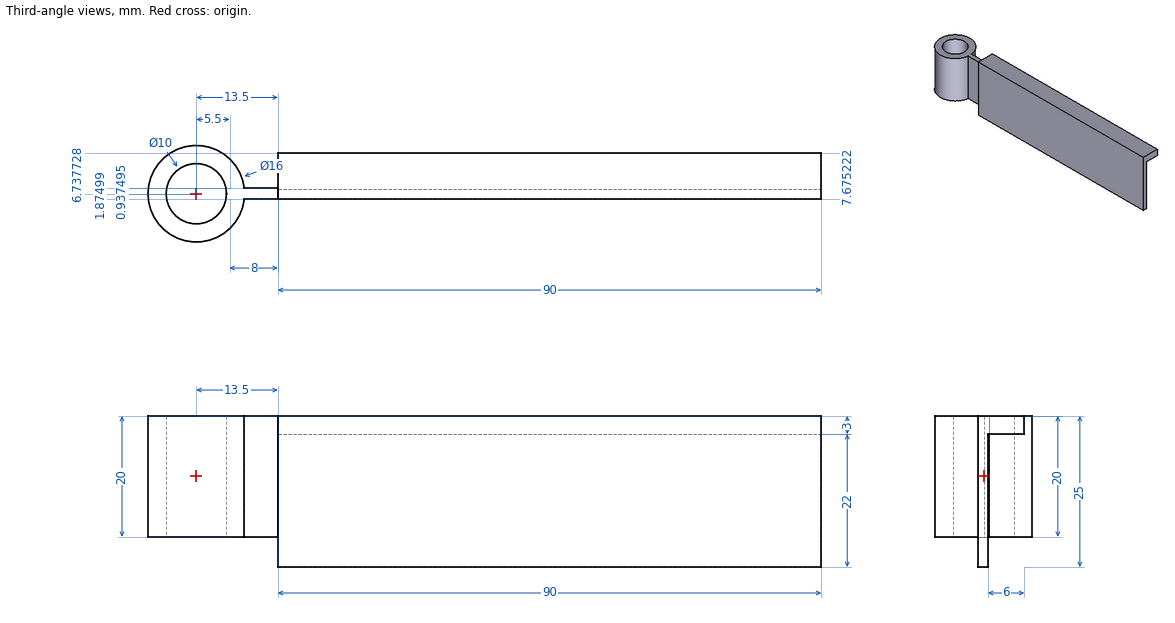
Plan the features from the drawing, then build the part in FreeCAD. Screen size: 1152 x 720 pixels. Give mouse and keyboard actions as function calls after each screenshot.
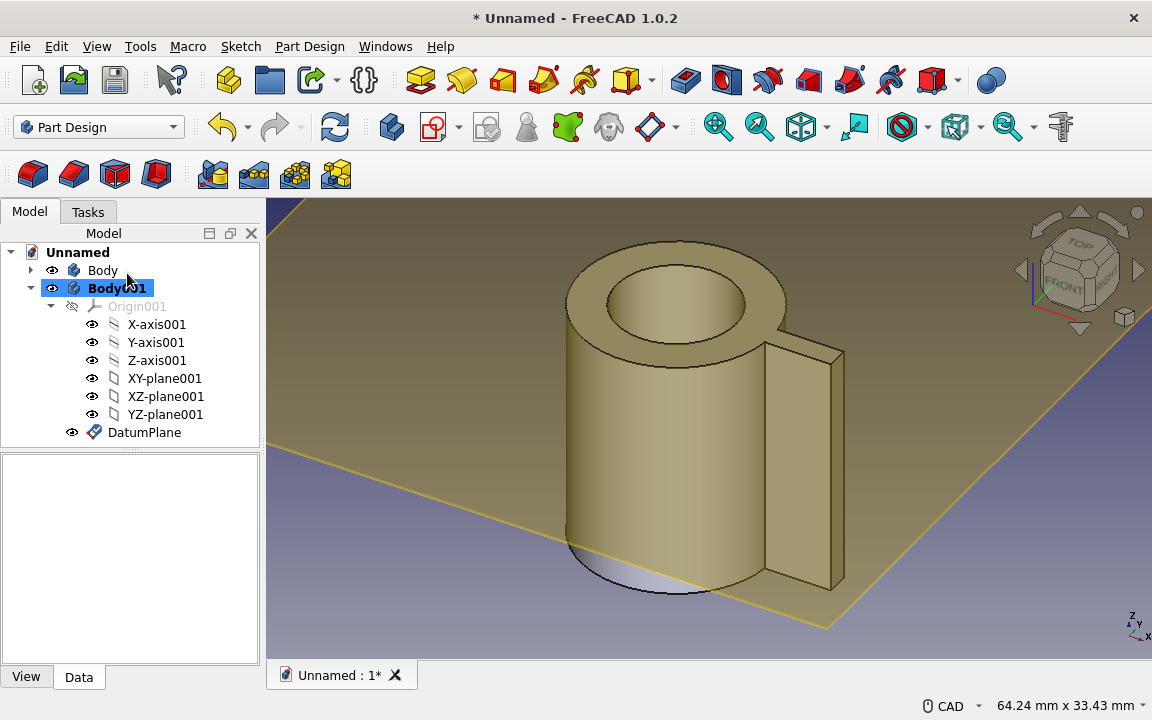
click(117, 432)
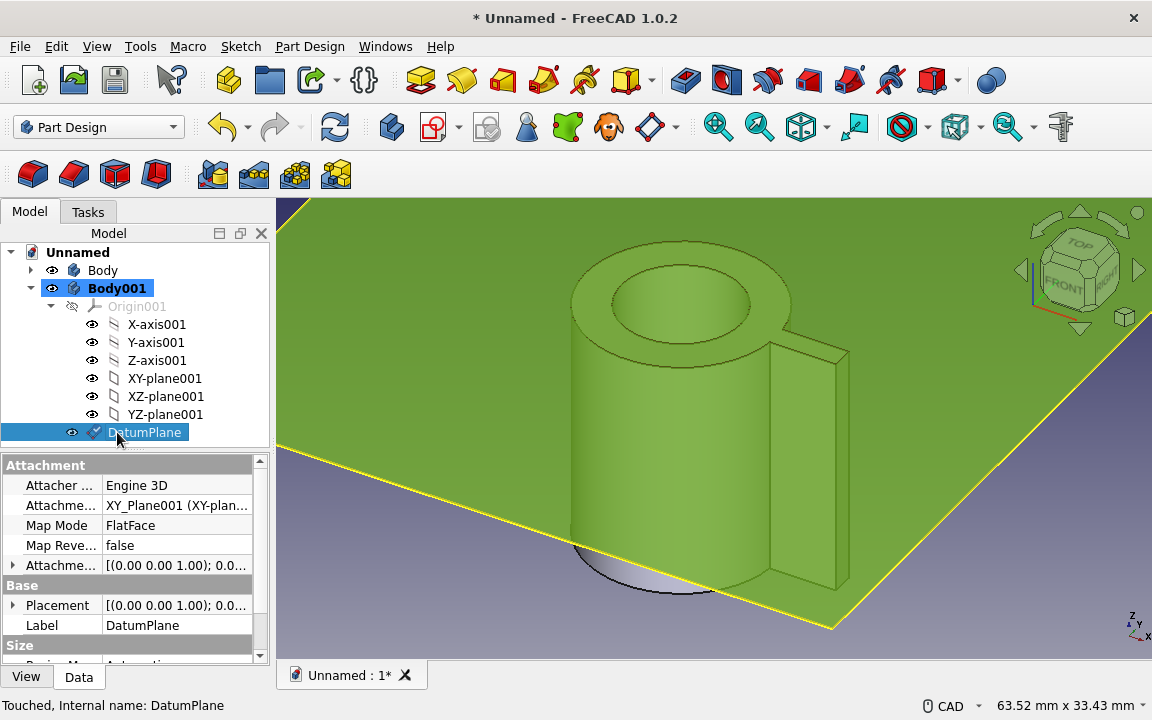
click(432, 128)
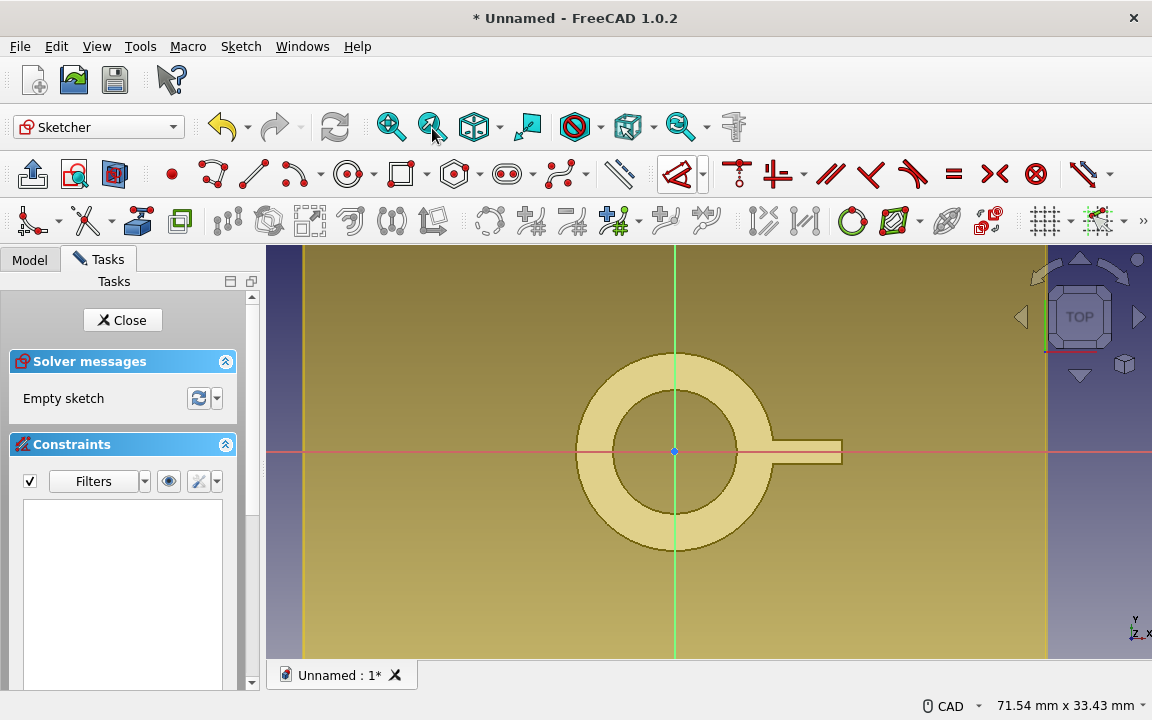
scroll(294, 473, down, 5)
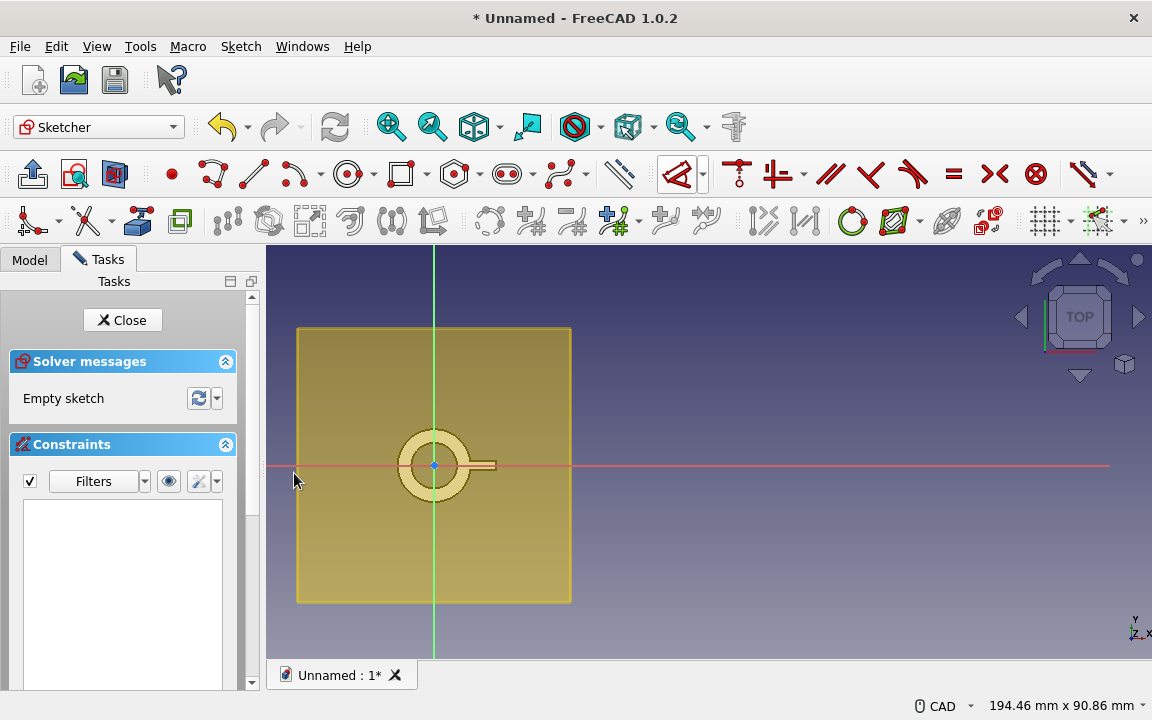
click(400, 174)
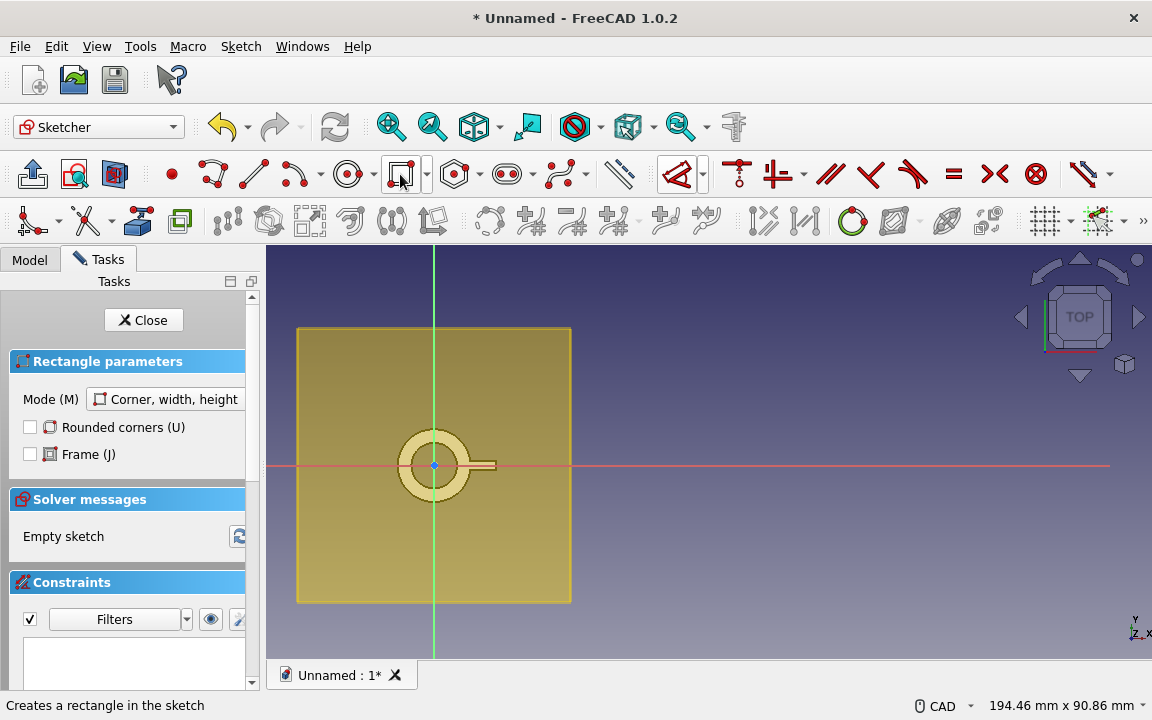
click(496, 435)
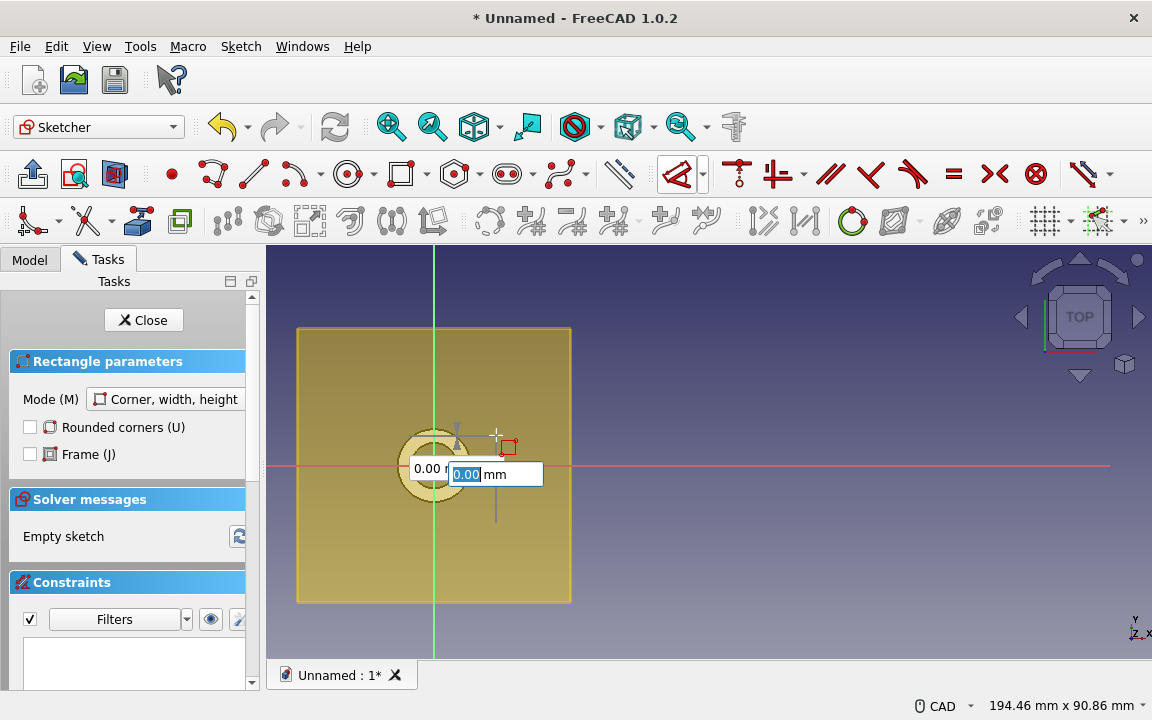
scroll(906, 470, up, 7)
move(903, 468)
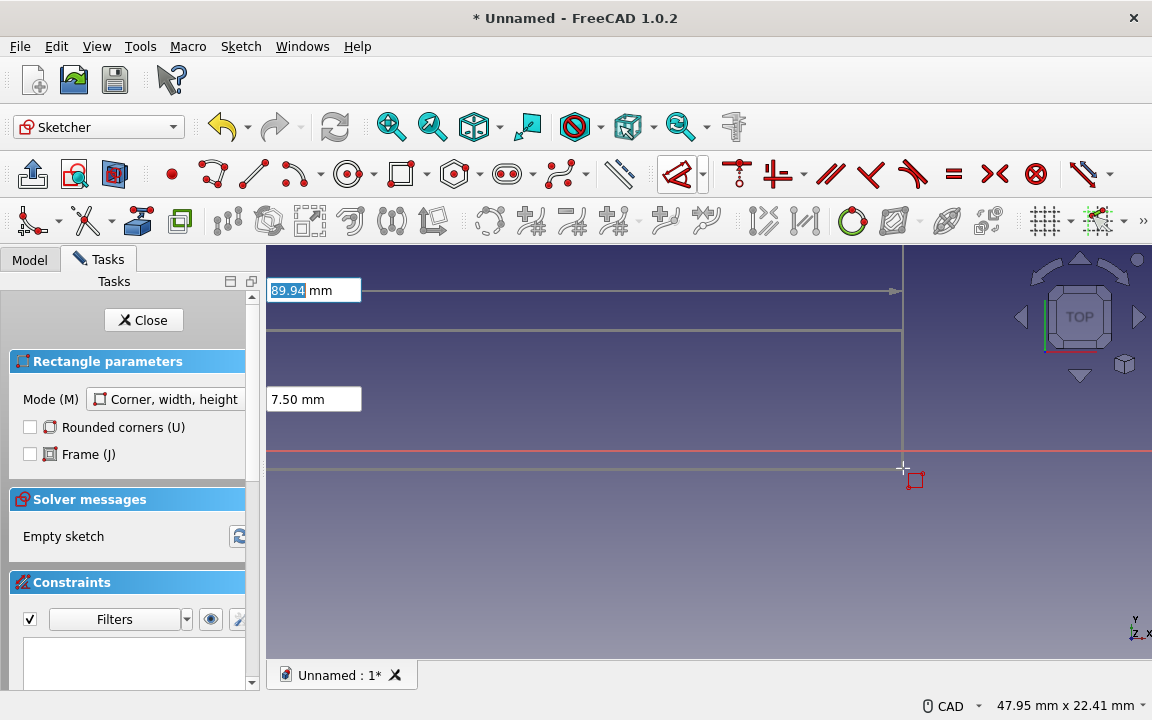
text(90)
key(Tab)
text(7.675222)
key(Return)
key(Escape)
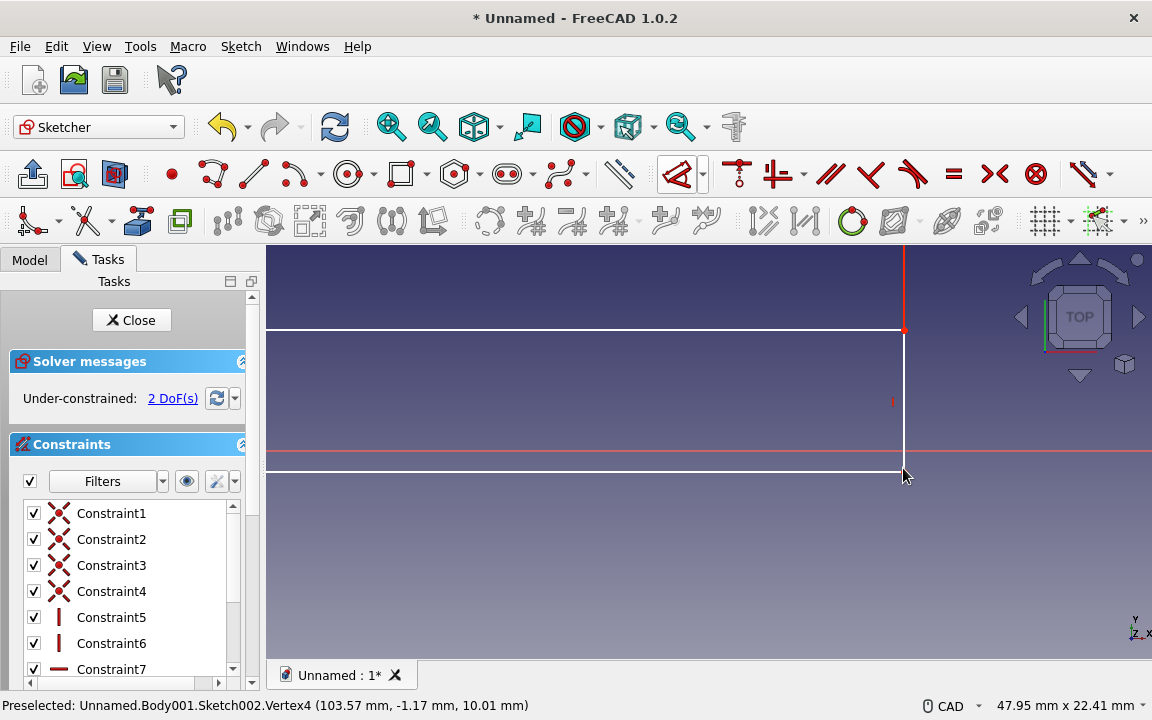
scroll(868, 470, down, 7)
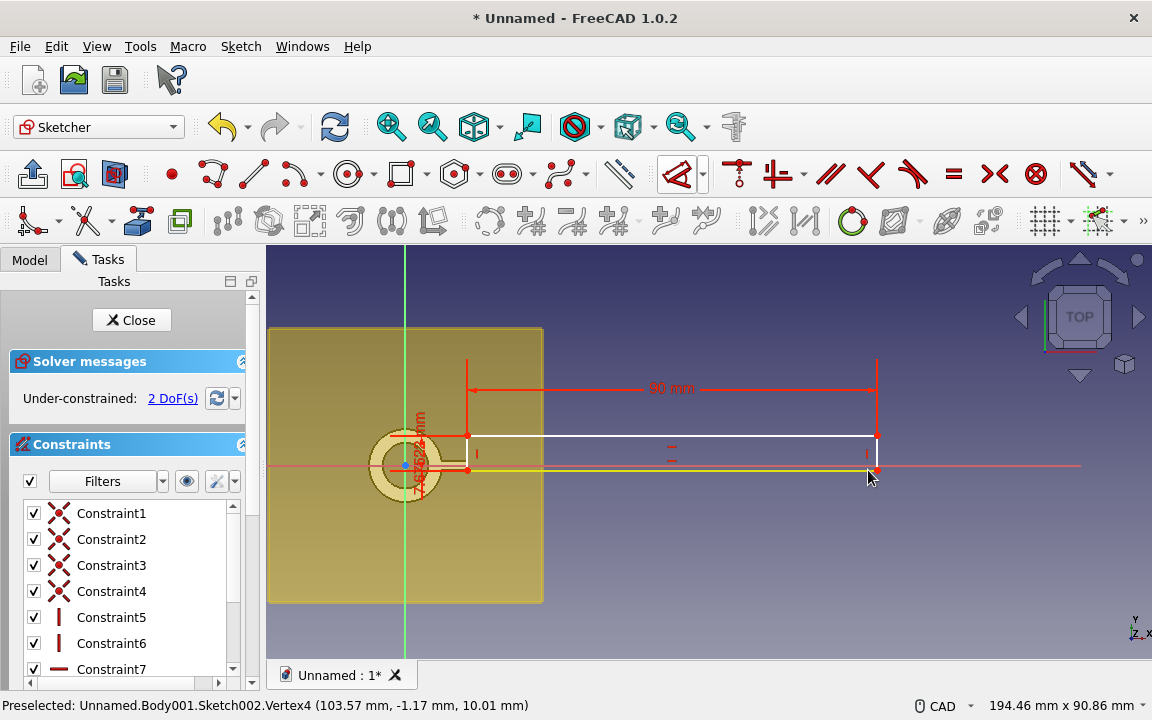
click(467, 436)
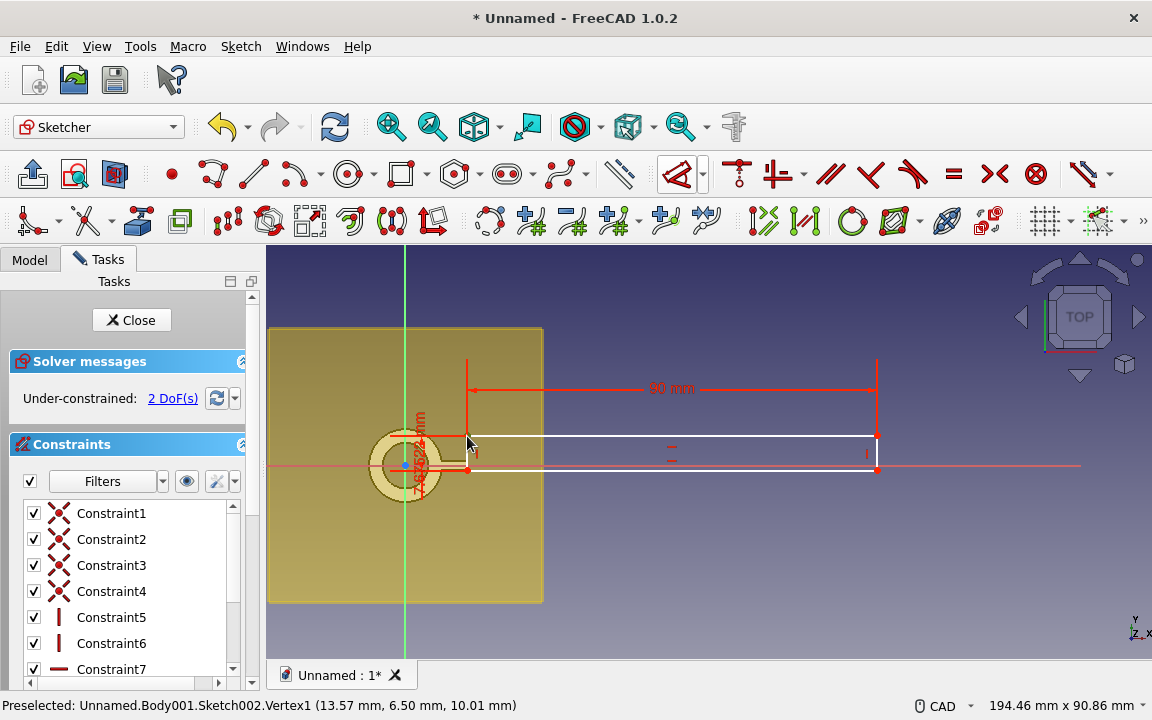
click(702, 174)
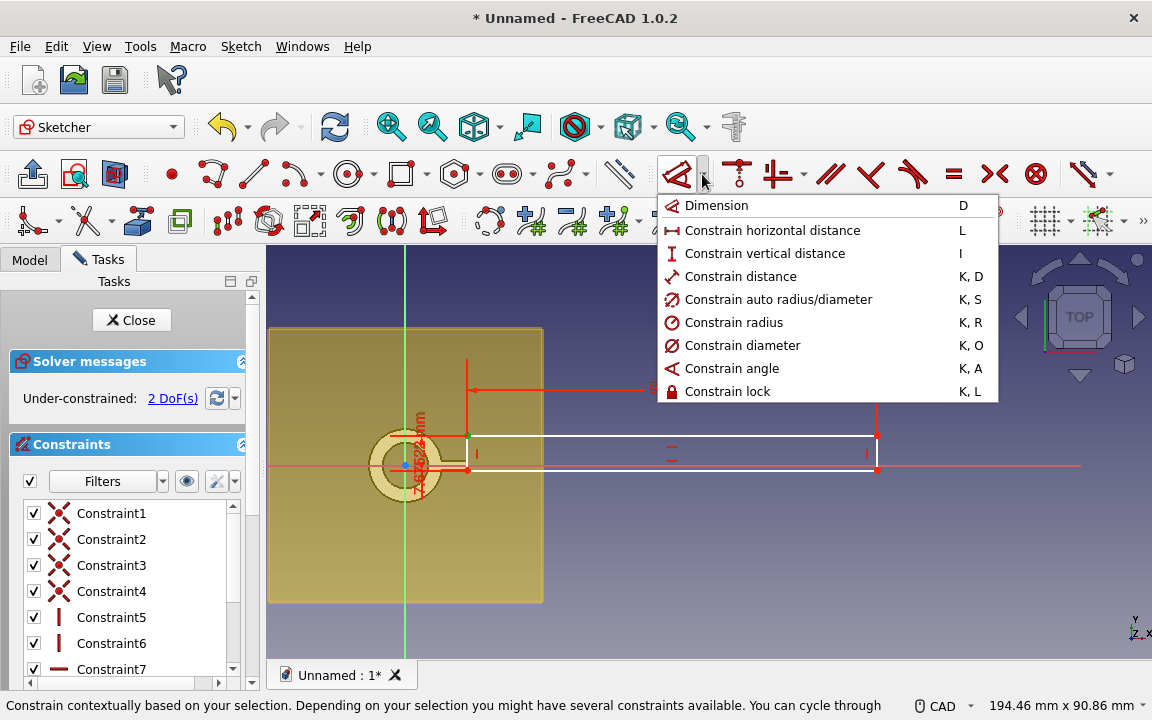
click(828, 230)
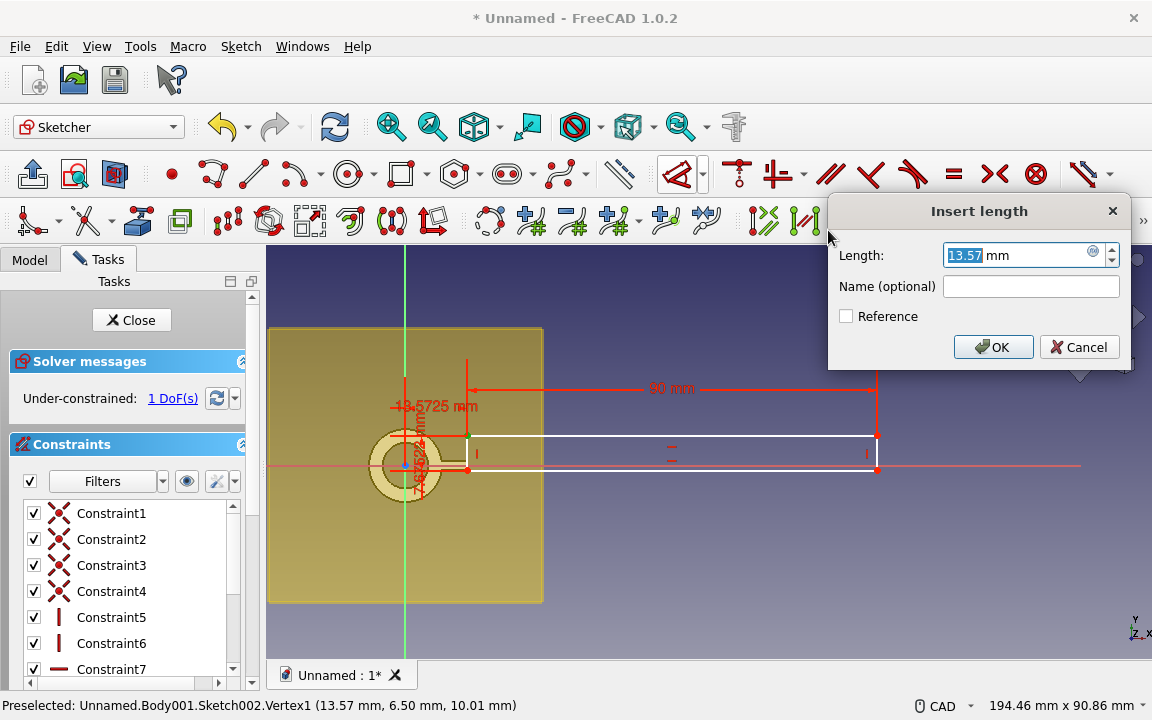
text(13.5)
key(Return)